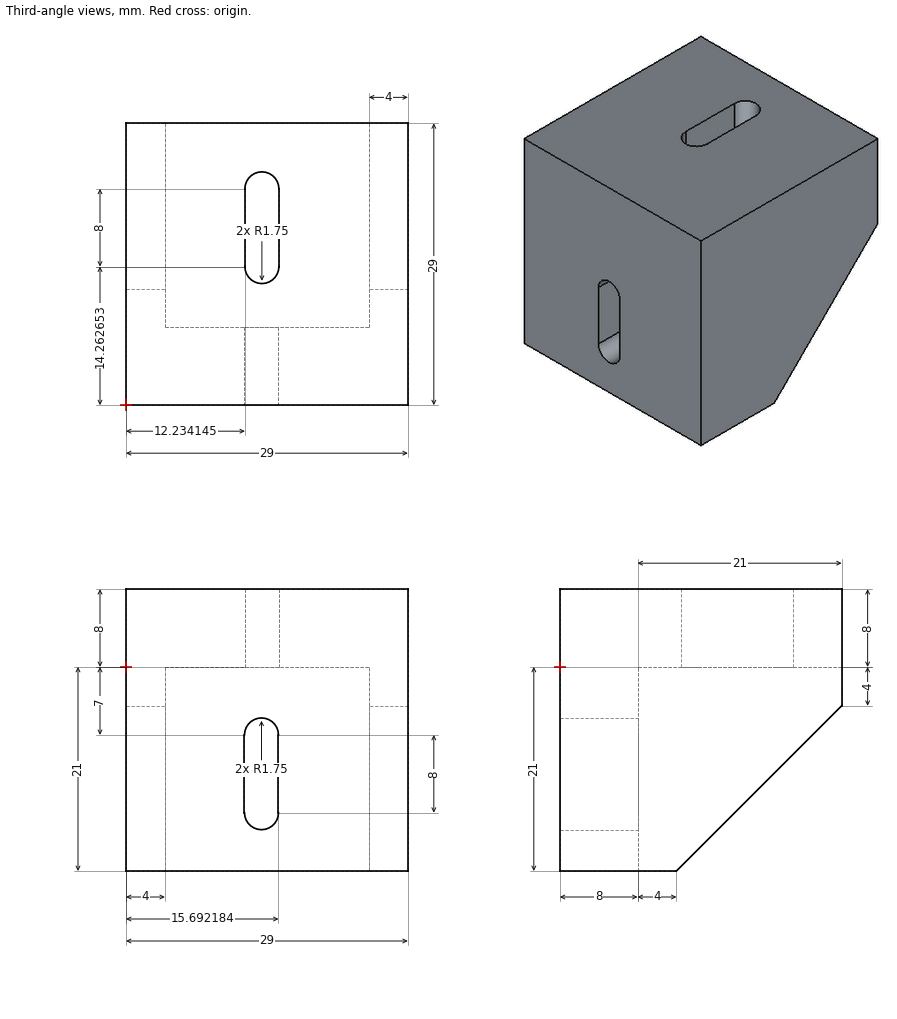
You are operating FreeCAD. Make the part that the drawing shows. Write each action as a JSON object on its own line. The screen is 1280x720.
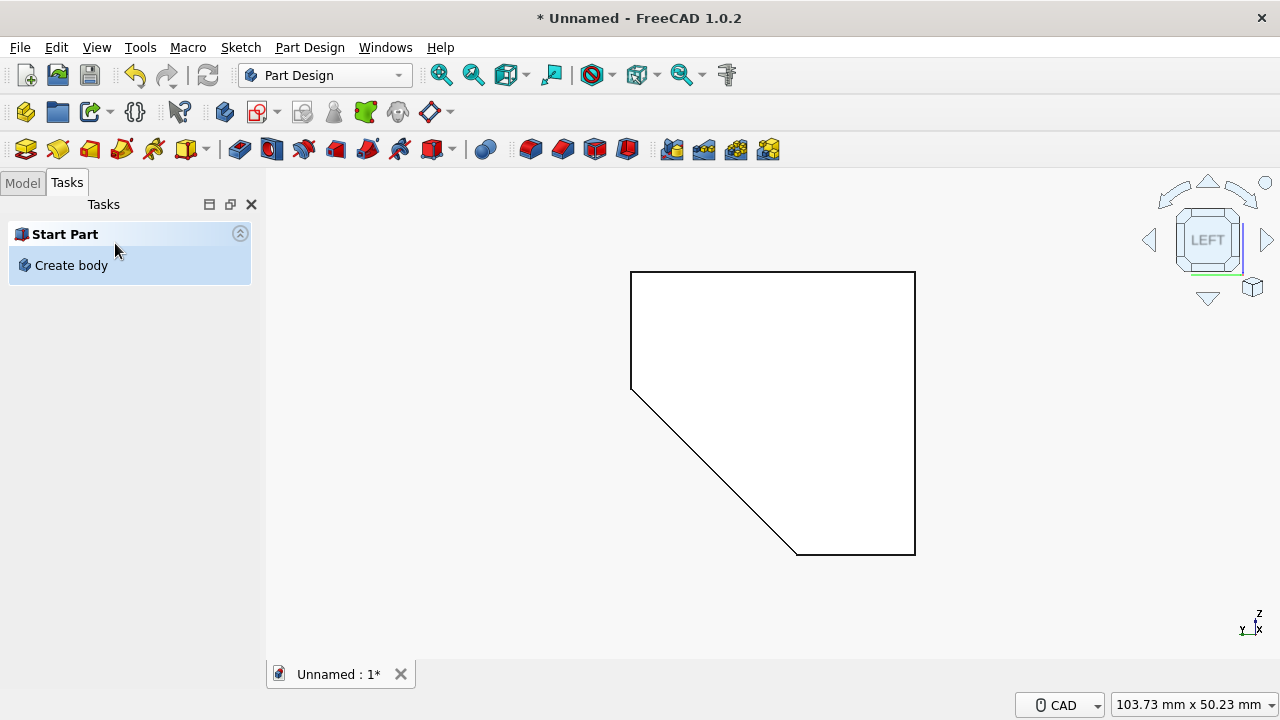
{"action": "key", "text": "0"}